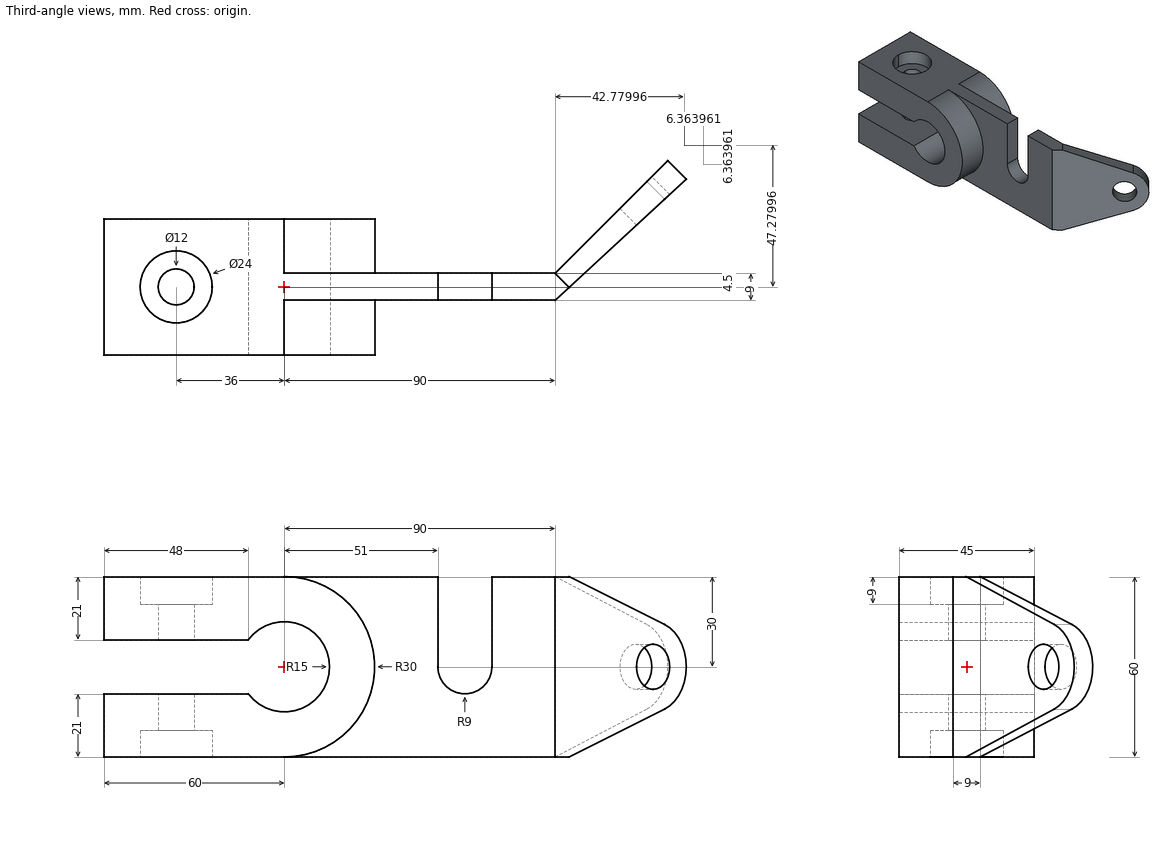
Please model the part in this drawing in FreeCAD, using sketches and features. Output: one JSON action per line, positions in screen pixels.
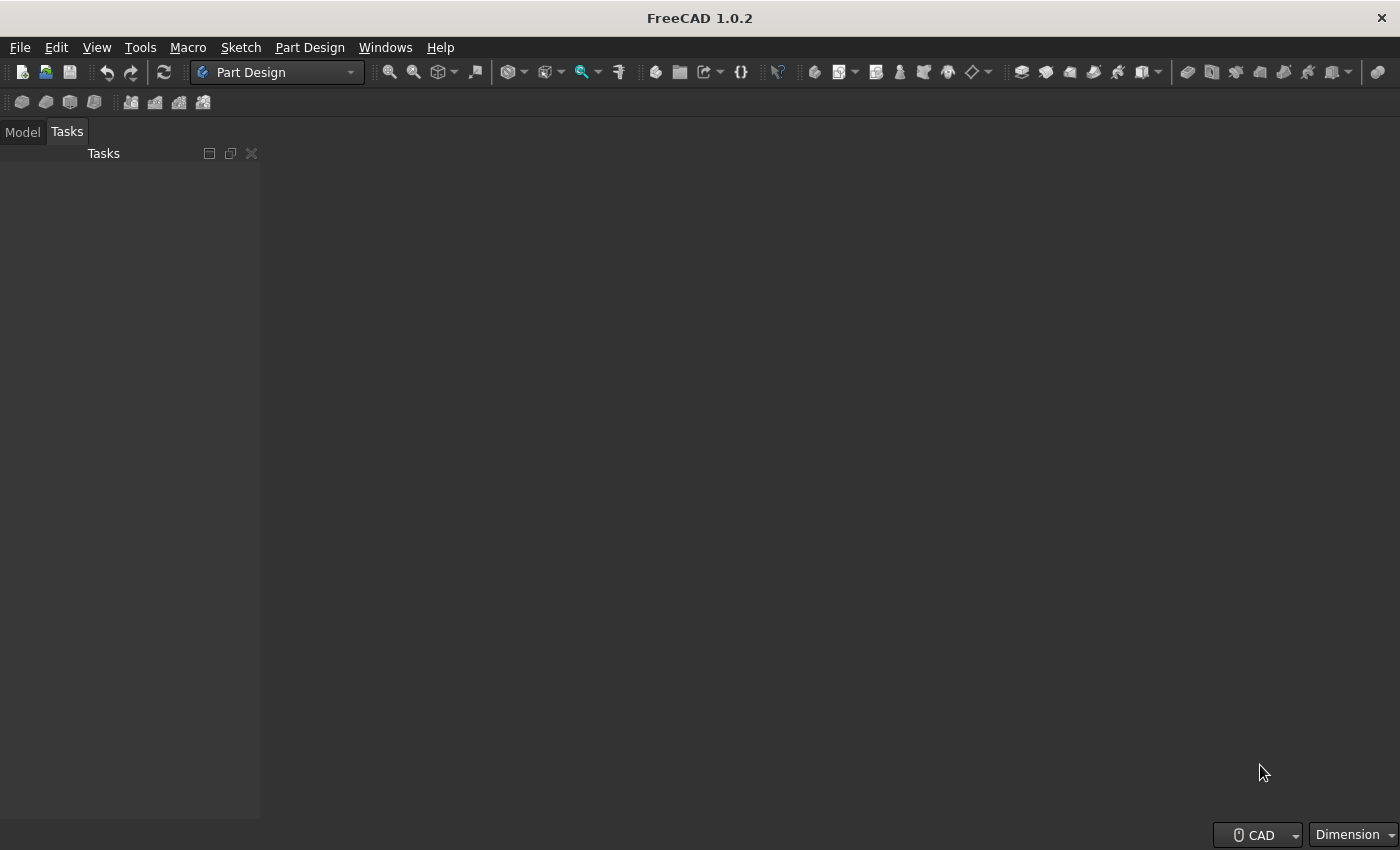
{"action": "left_click", "coordinate": [22, 72]}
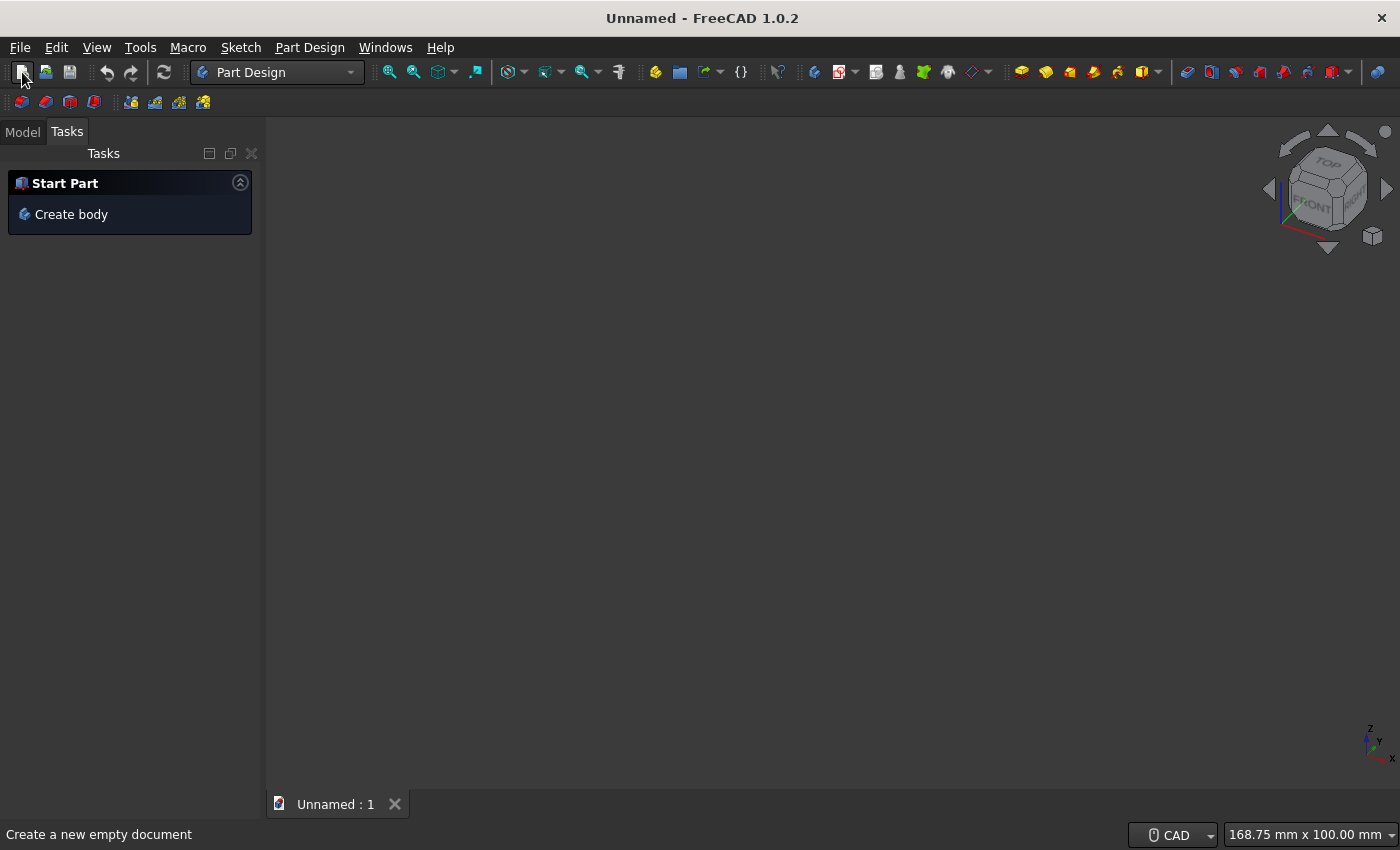
{"action": "left_click", "coordinate": [840, 72]}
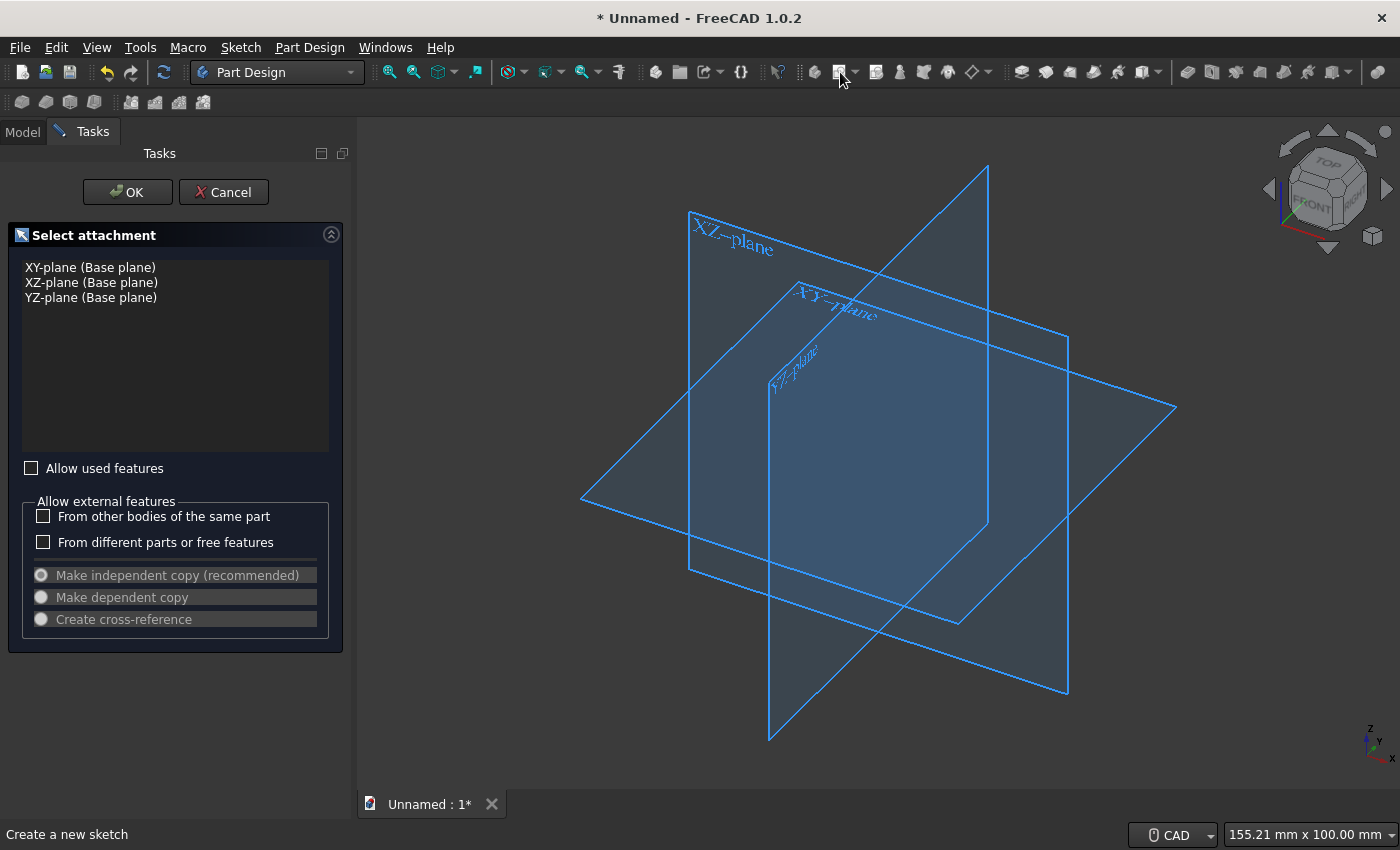
{"action": "left_click", "coordinate": [82, 282]}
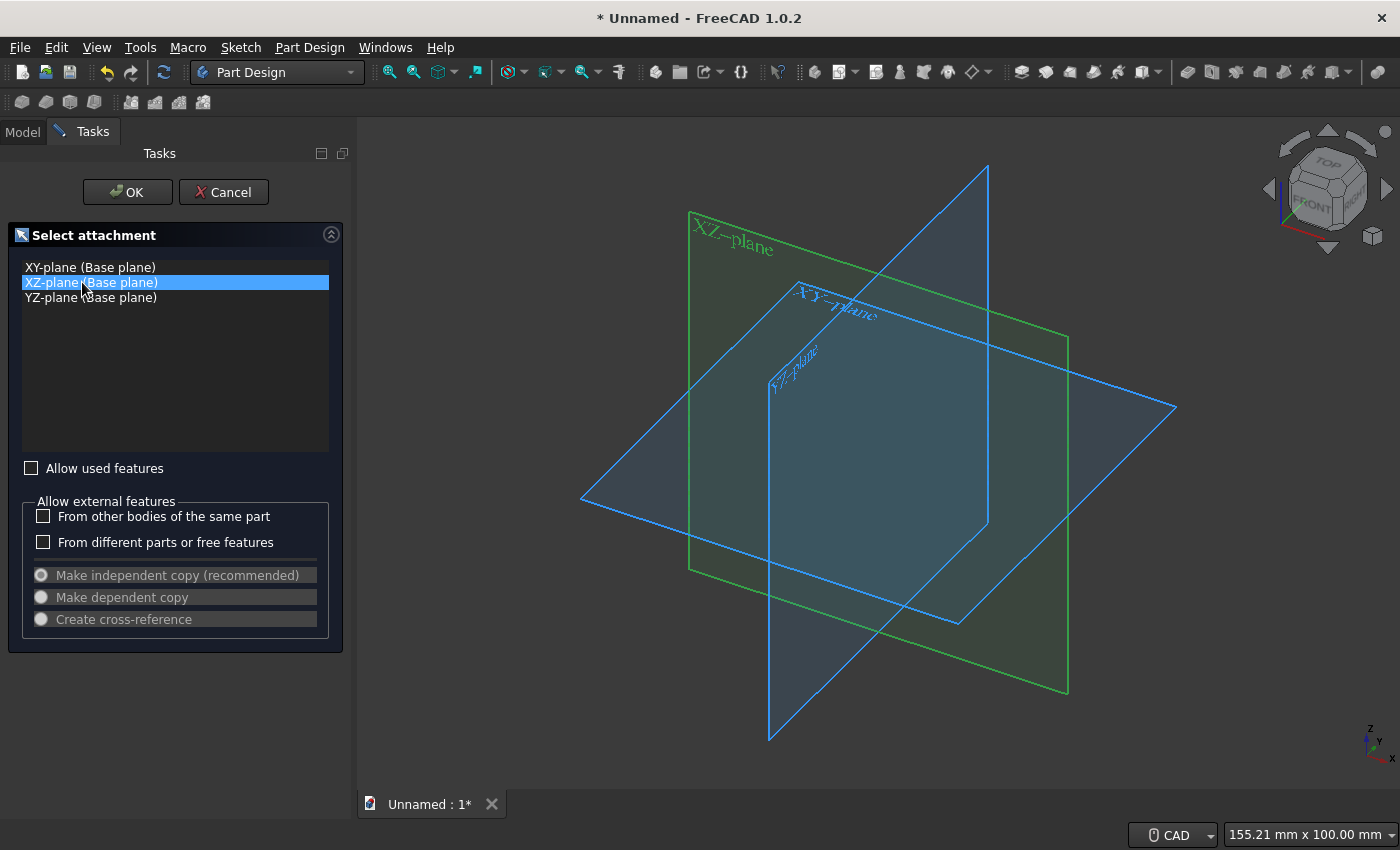
{"action": "left_click", "coordinate": [128, 192]}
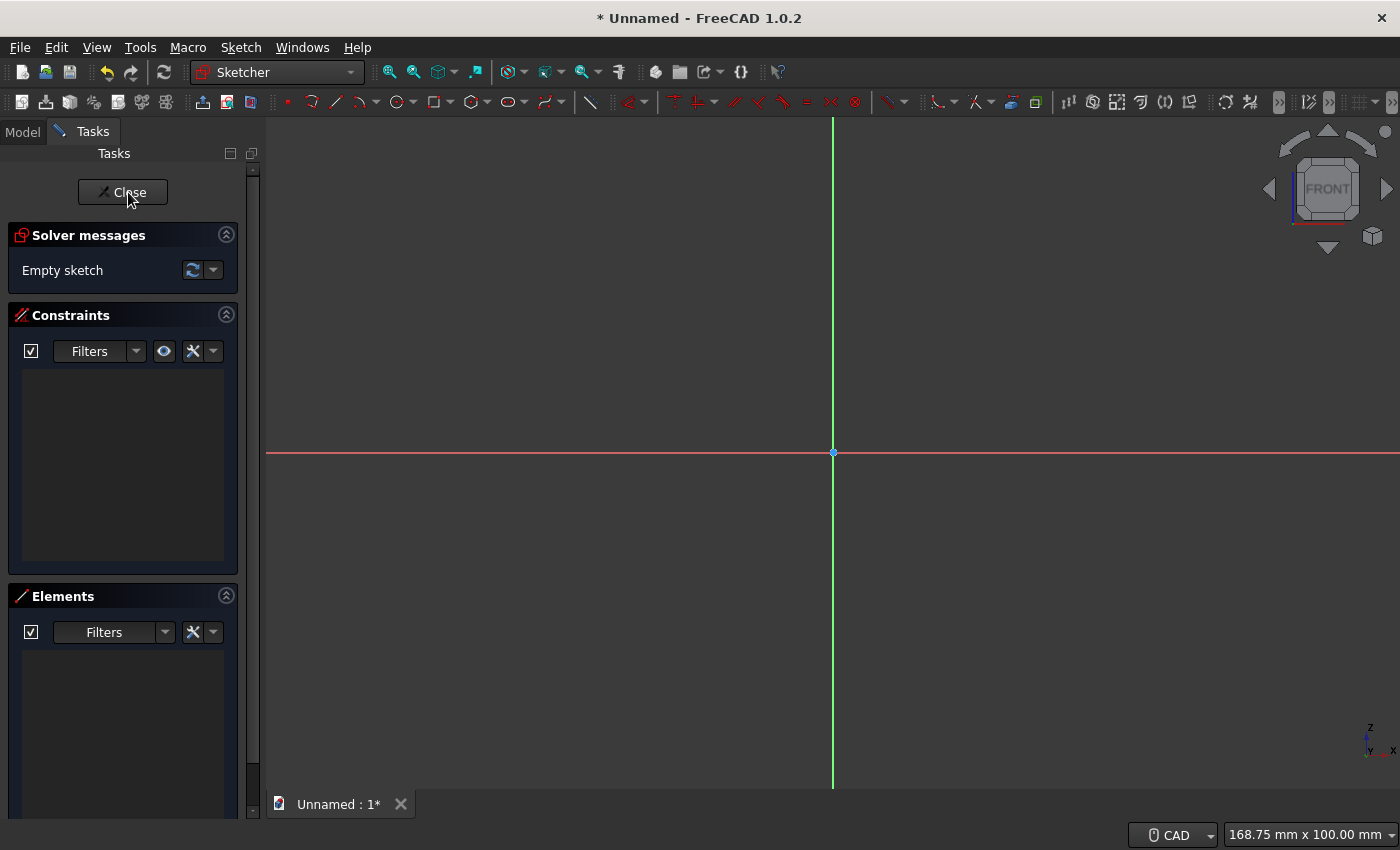
{"action": "key", "text": "g m"}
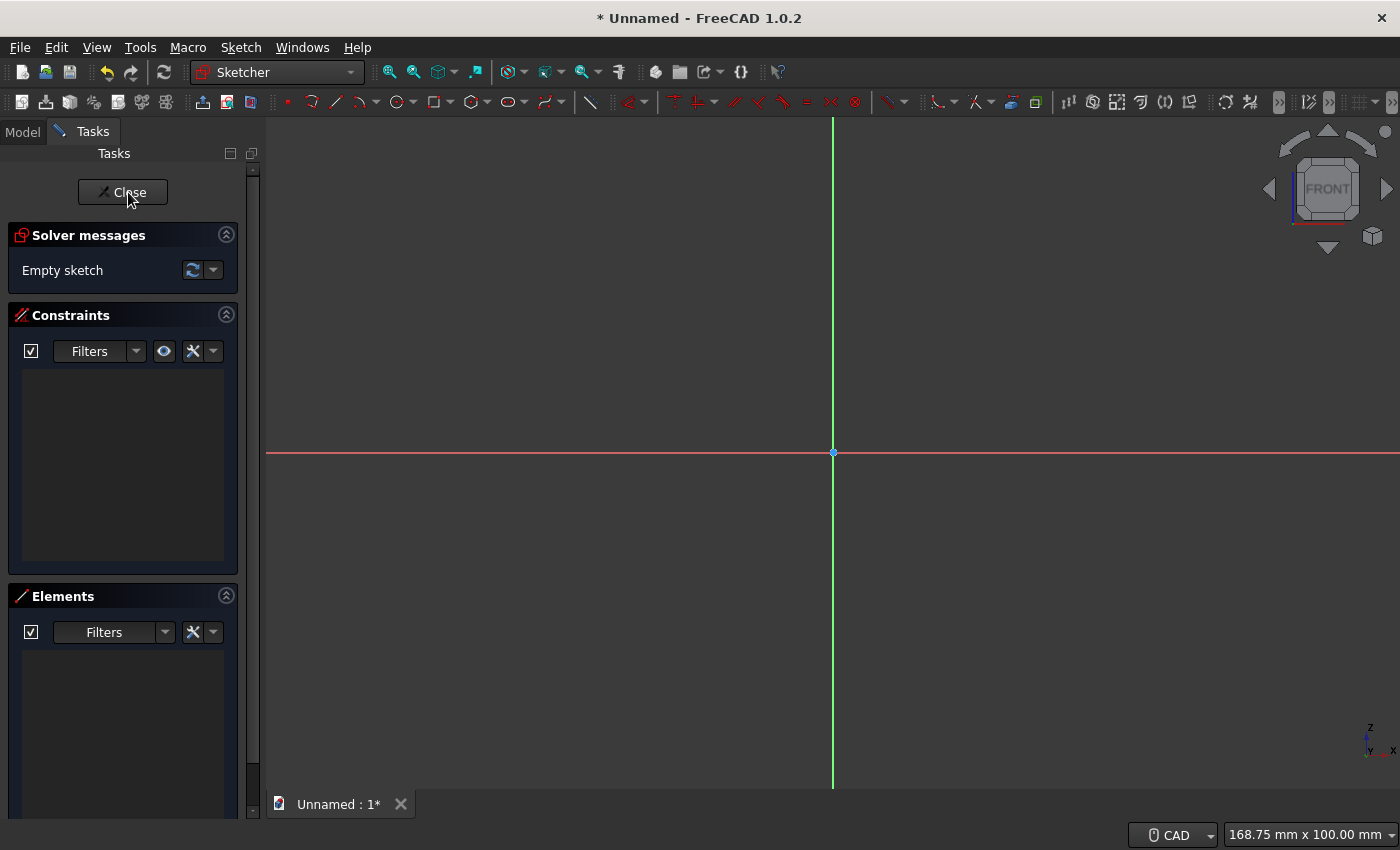
{"action": "left_click", "coordinate": [752, 393]}
{"action": "left_click", "coordinate": [430, 393]}
{"action": "left_click", "coordinate": [430, 251]}
{"action": "left_click", "coordinate": [833, 251]}
{"action": "right_click", "coordinate": [833, 251]}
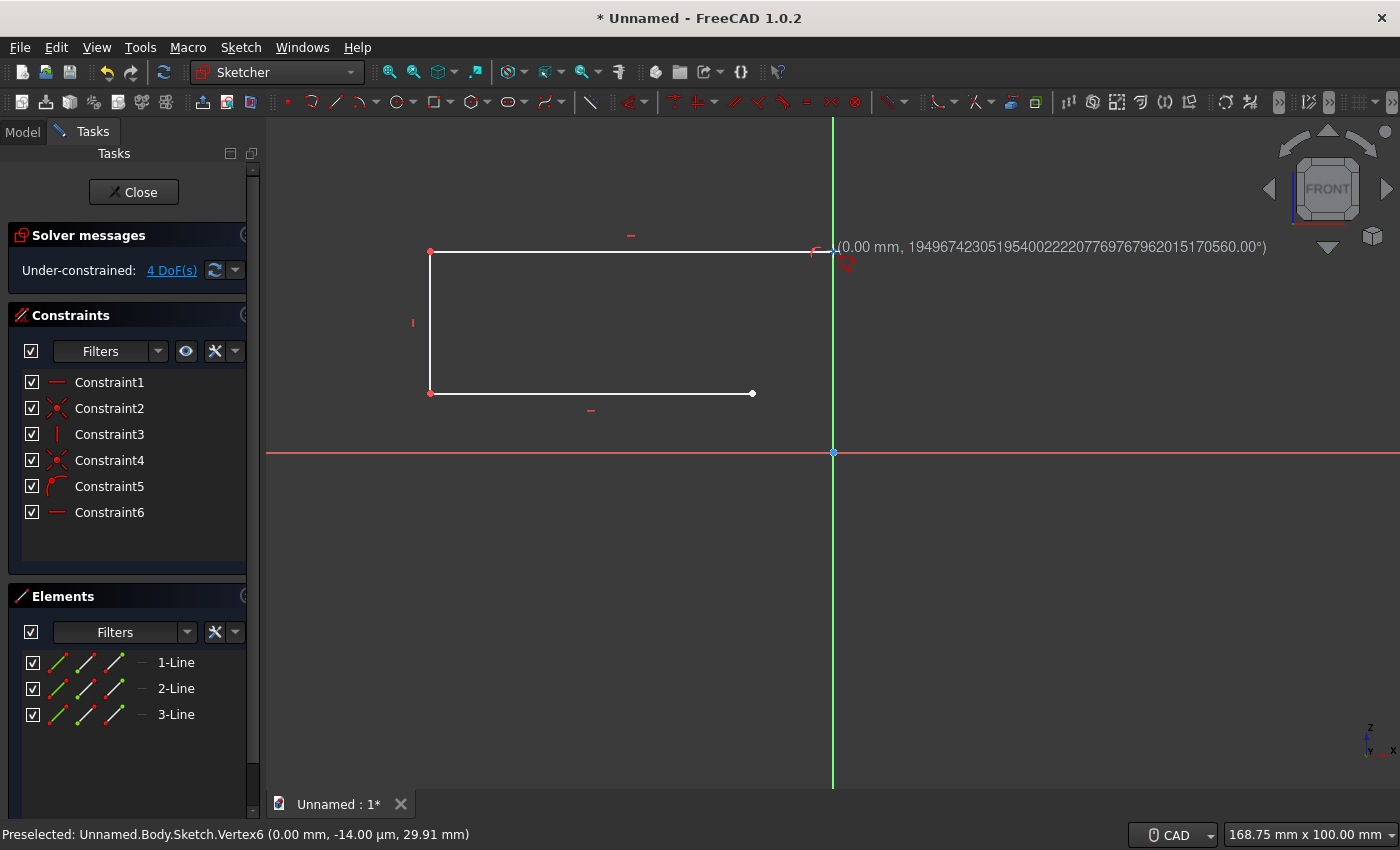
{"action": "left_click", "coordinate": [833, 655]}
{"action": "left_click", "coordinate": [430, 655]}
{"action": "left_click", "coordinate": [430, 513]}
{"action": "left_click", "coordinate": [752, 513]}
{"action": "right_click", "coordinate": [752, 513]}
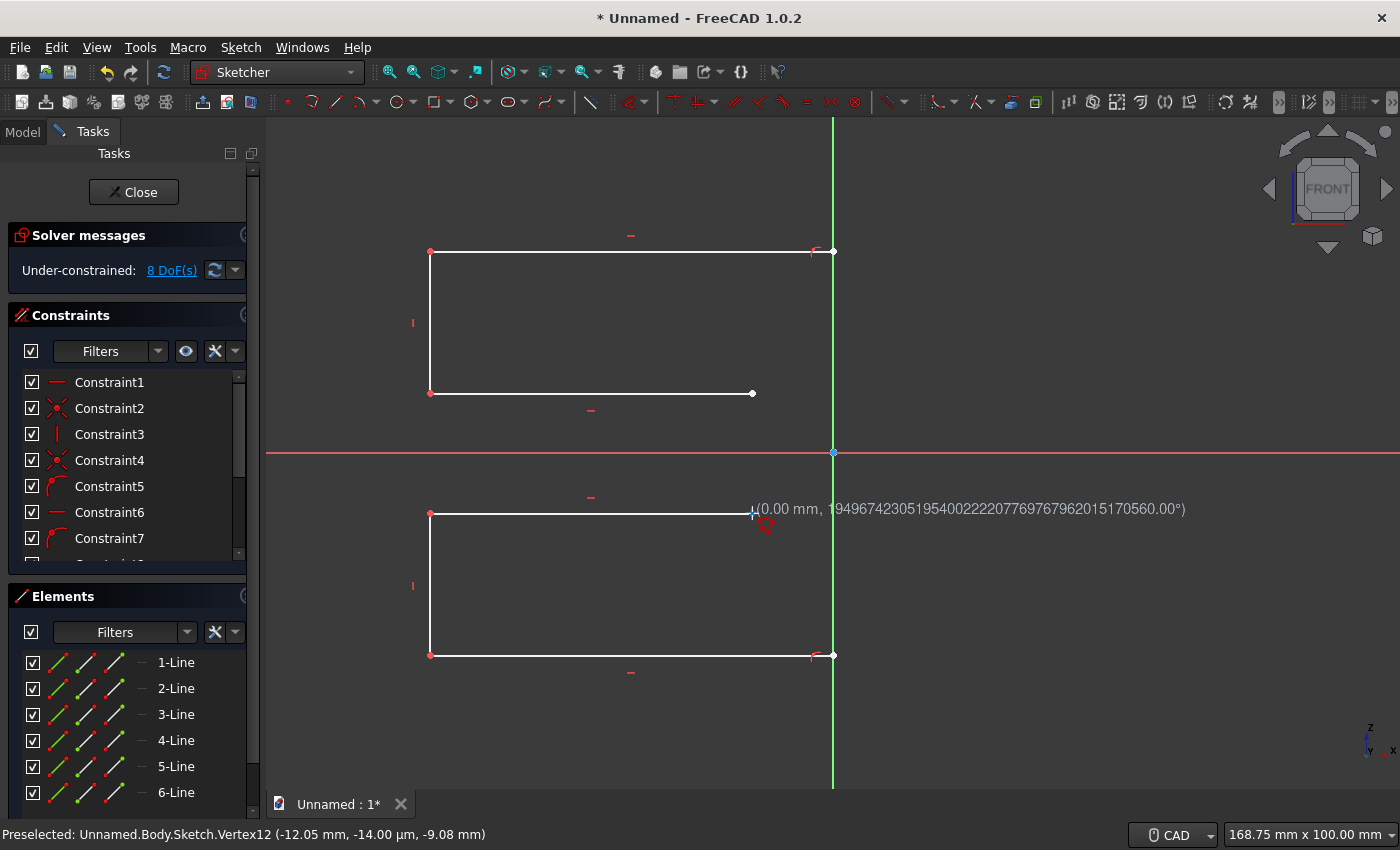
{"action": "key", "text": "g 3 a"}